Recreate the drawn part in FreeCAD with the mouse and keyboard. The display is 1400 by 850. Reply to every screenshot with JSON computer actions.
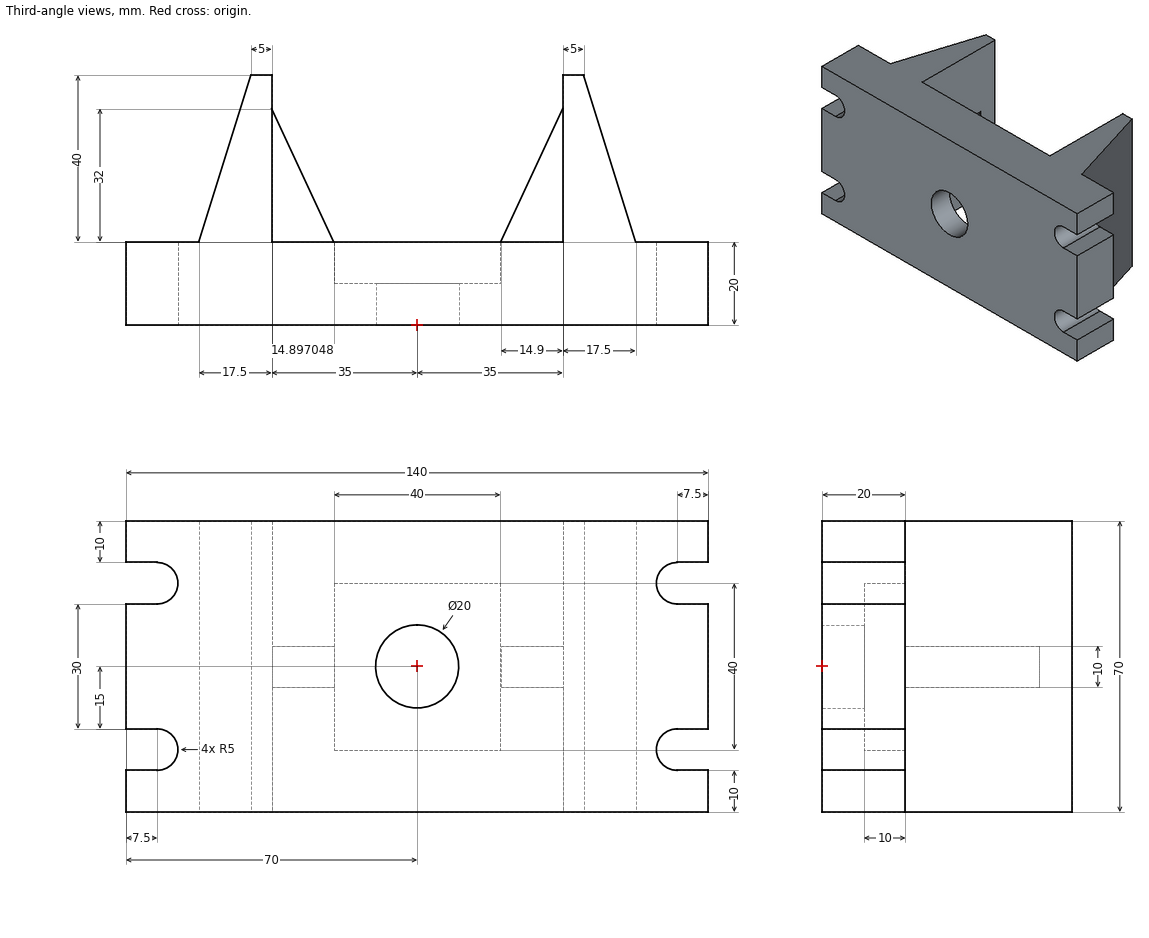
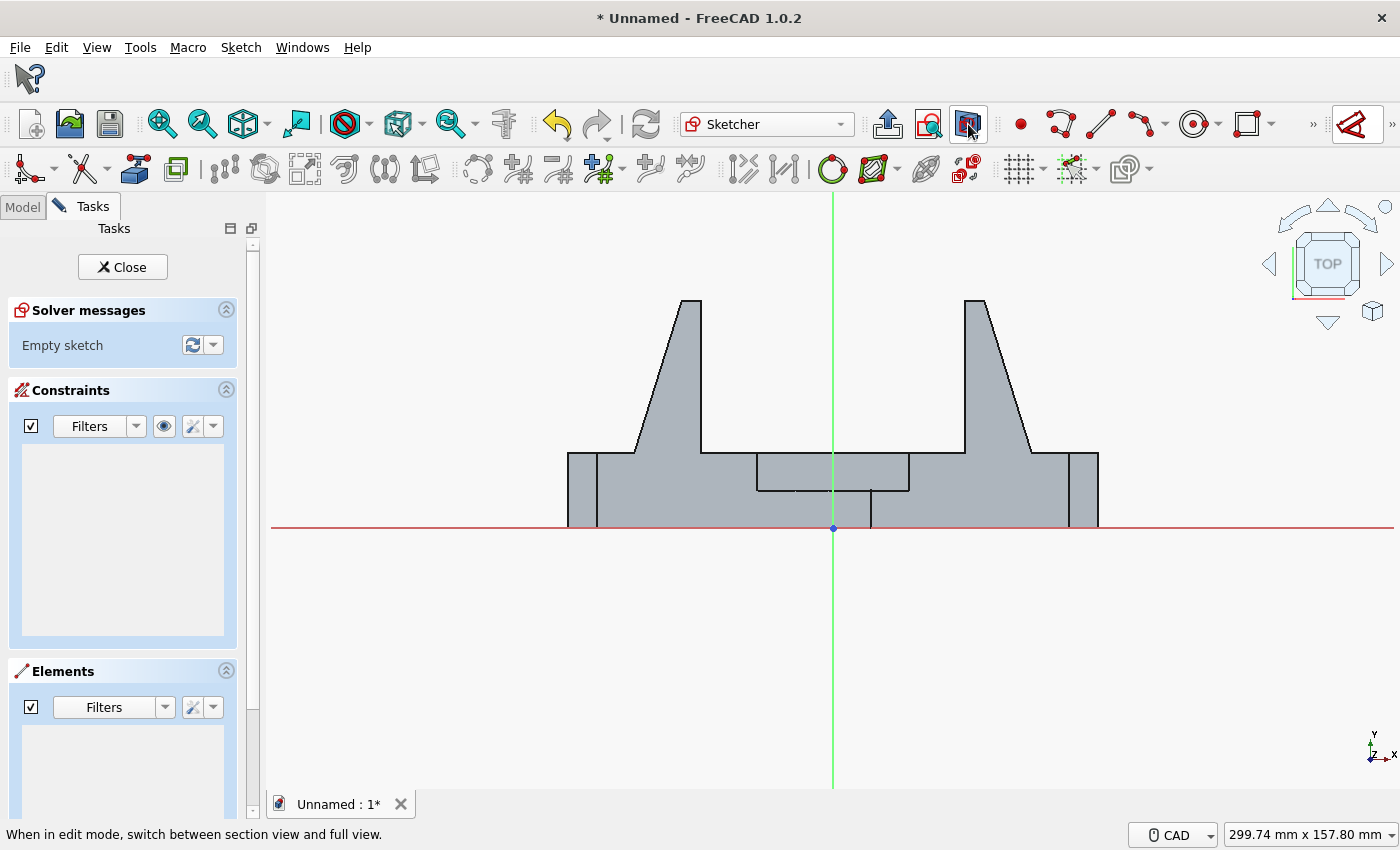
{"action": "scroll", "coordinate": [916, 356], "scroll_direction": "up", "scroll_amount": 3}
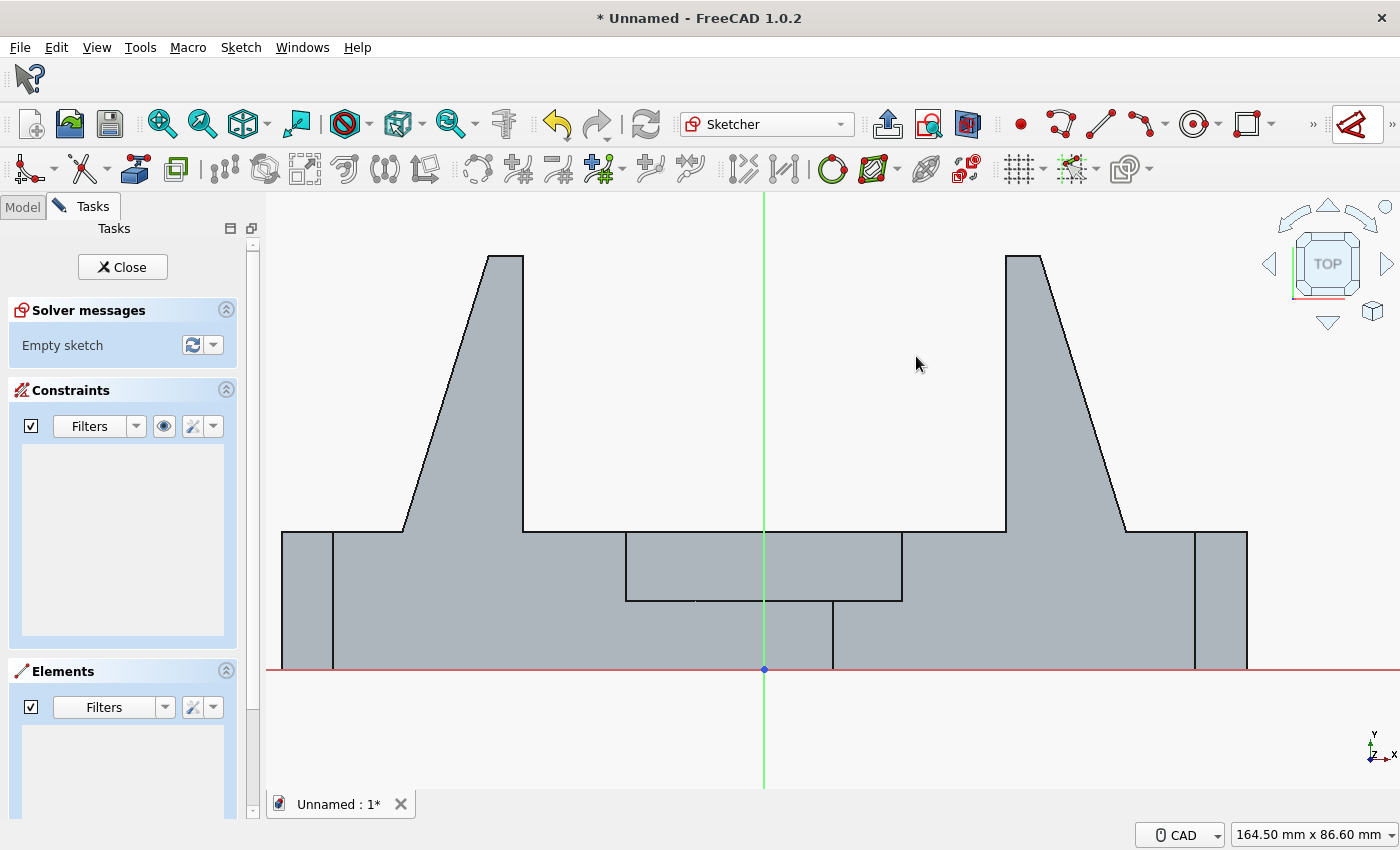
{"action": "left_click", "coordinate": [1062, 124]}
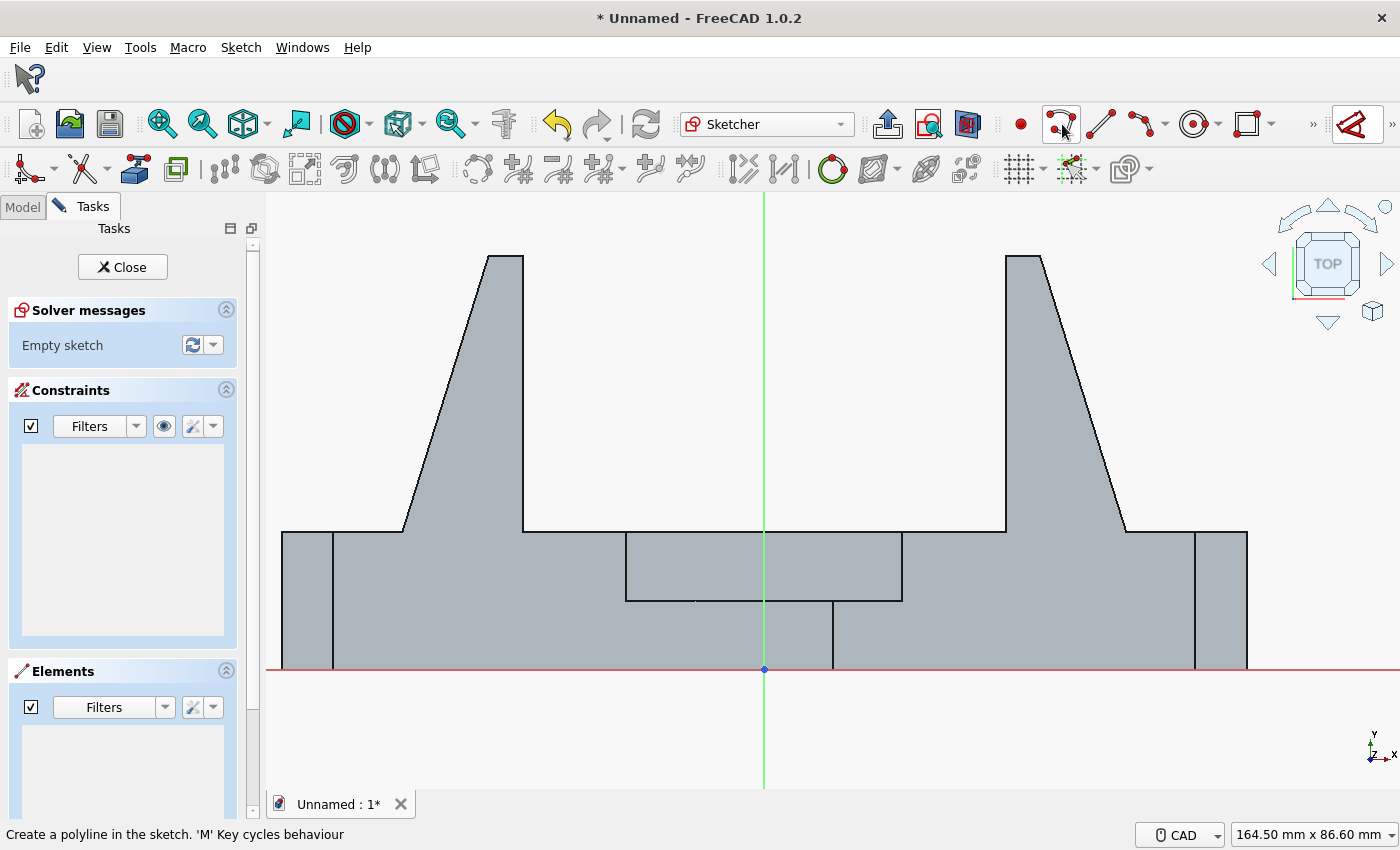
{"action": "left_click", "coordinate": [626, 532]}
{"action": "left_click", "coordinate": [523, 311]}
{"action": "left_click", "coordinate": [523, 532]}
{"action": "left_click", "coordinate": [626, 533]}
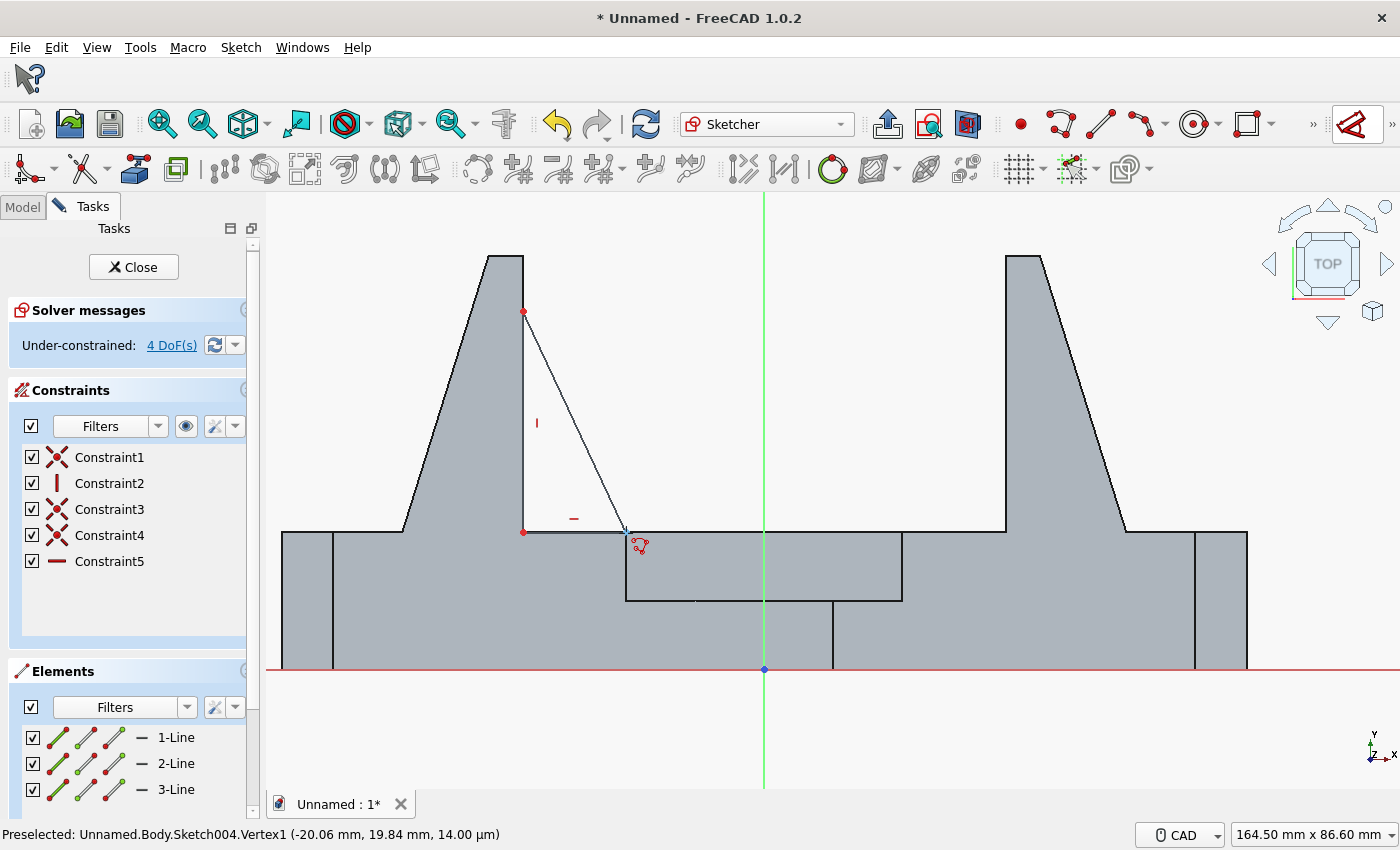
{"action": "left_click", "coordinate": [903, 532]}
{"action": "left_click", "coordinate": [1006, 532]}
{"action": "left_click", "coordinate": [1006, 311]}
{"action": "left_click", "coordinate": [903, 533]}
{"action": "key", "text": "Escape"}
{"action": "key", "text": "Escape"}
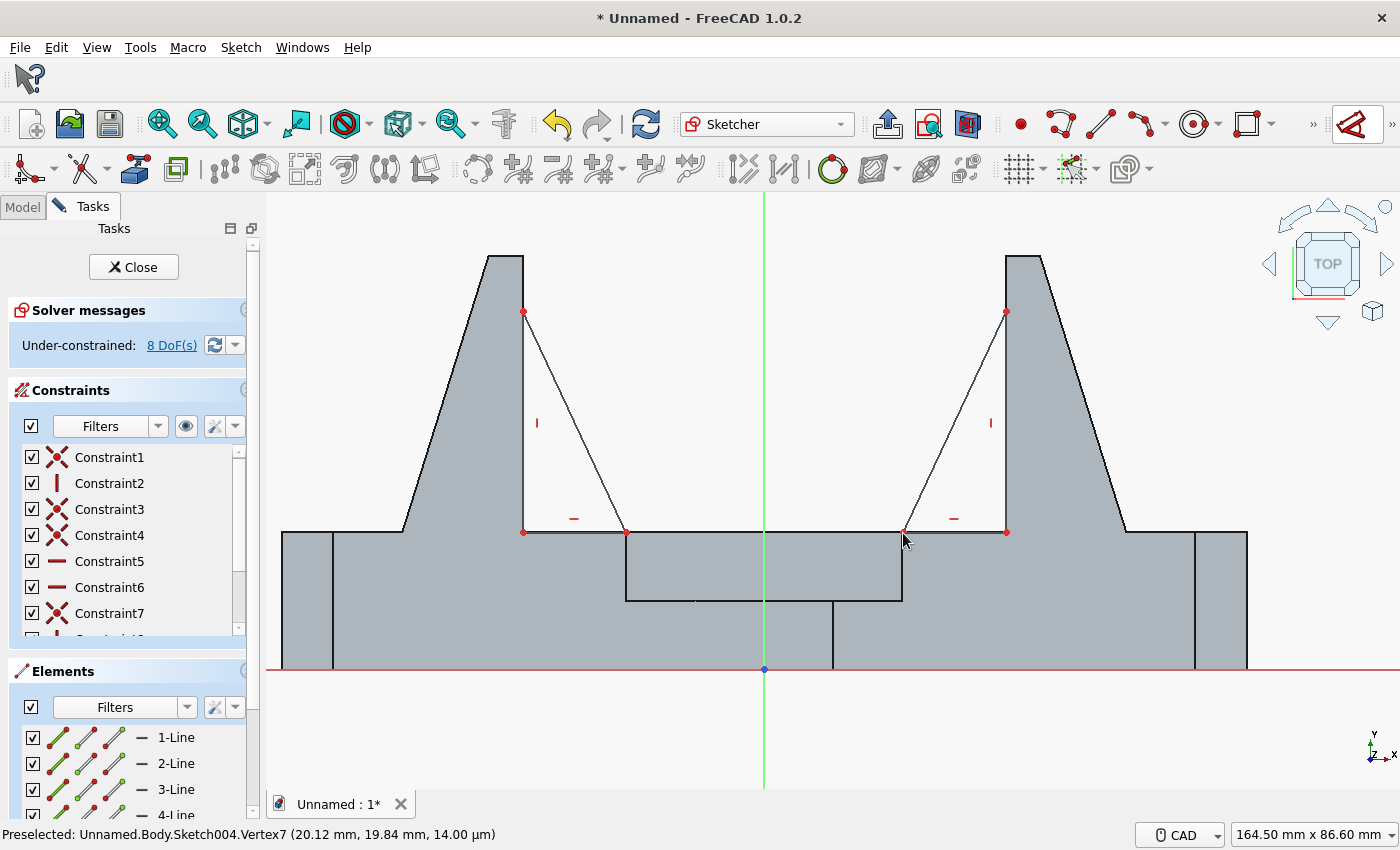
{"action": "left_click", "coordinate": [523, 378]}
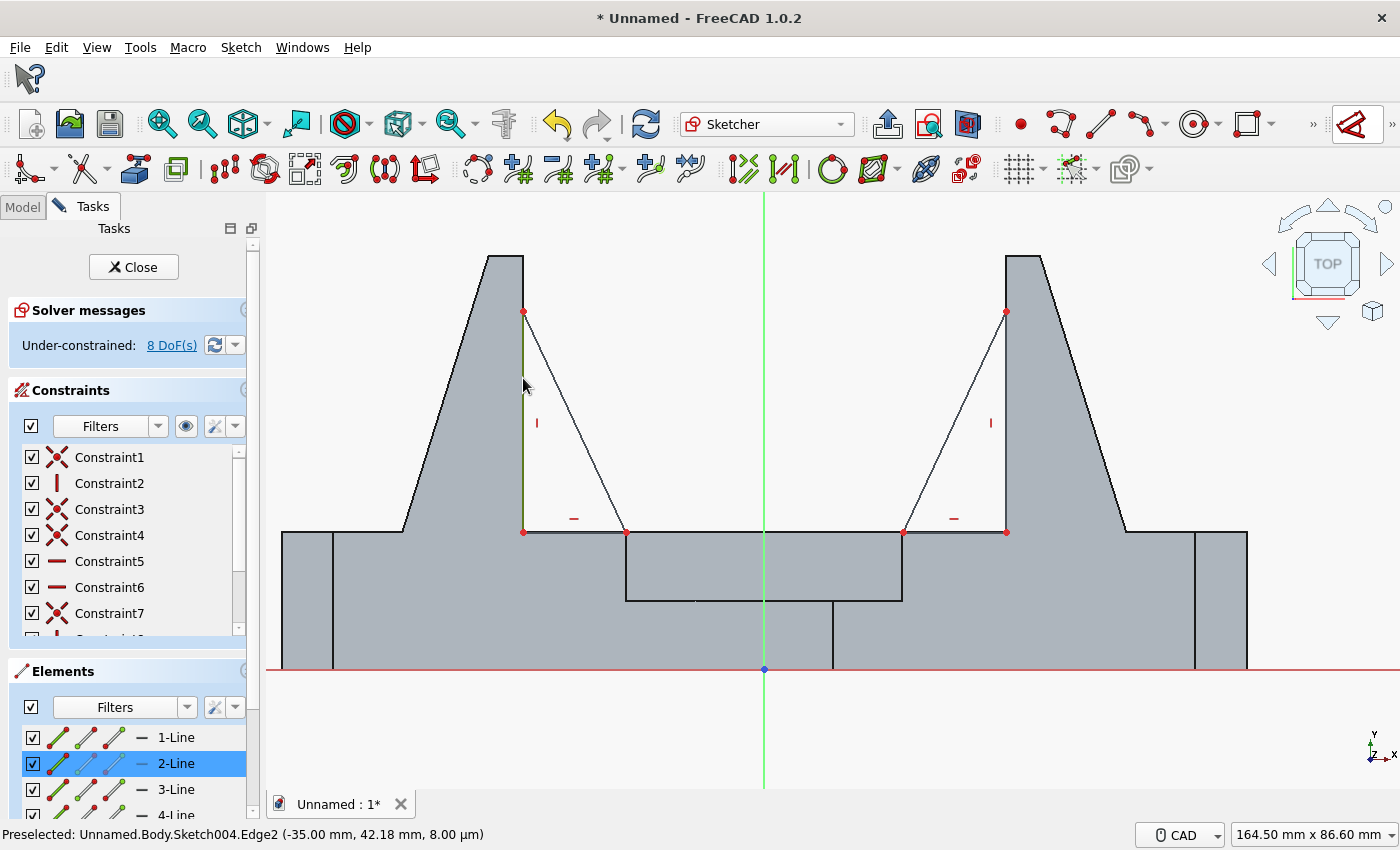
{"action": "key", "text": "i"}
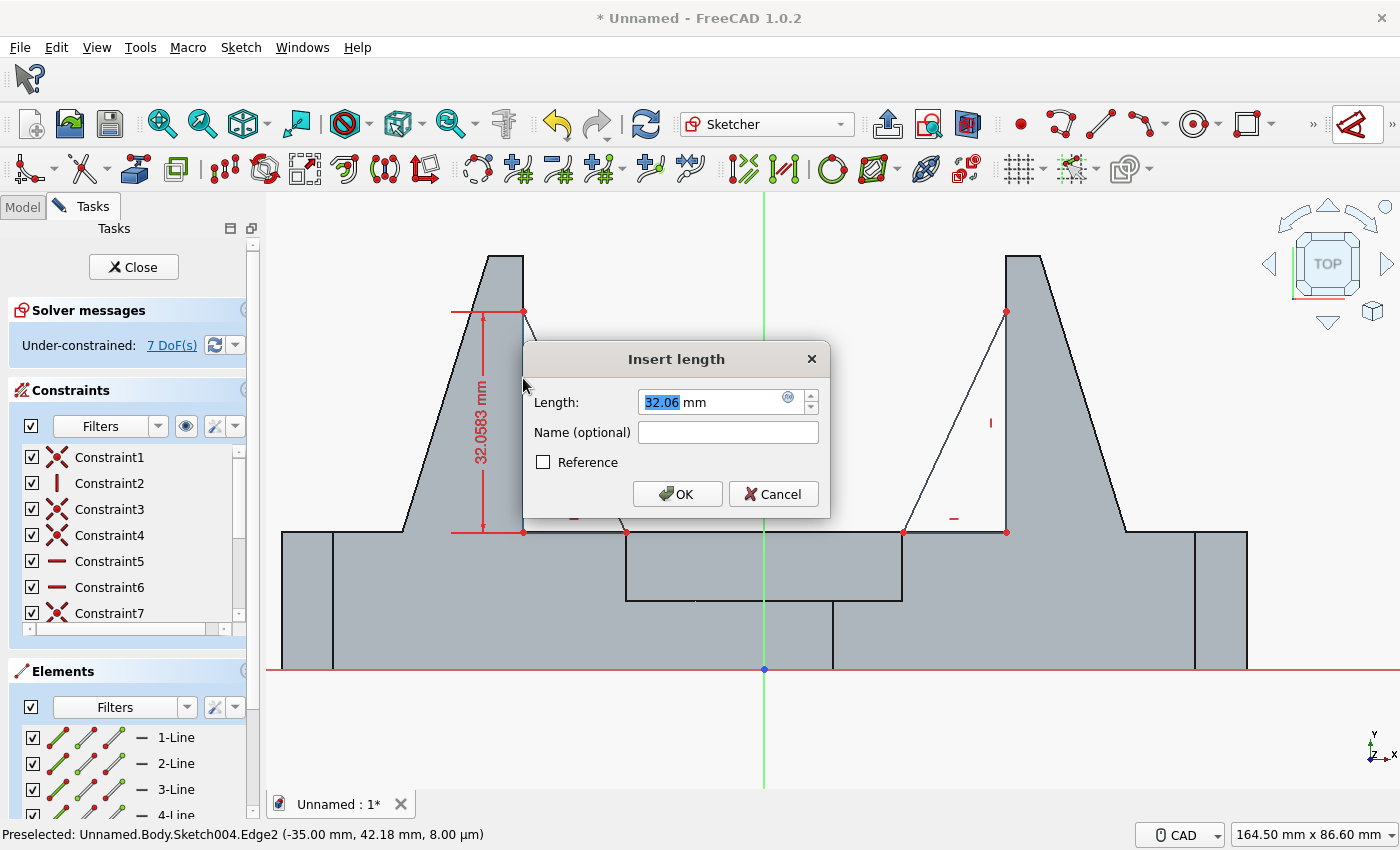
{"action": "type", "text": "32"}
{"action": "key", "text": "Return"}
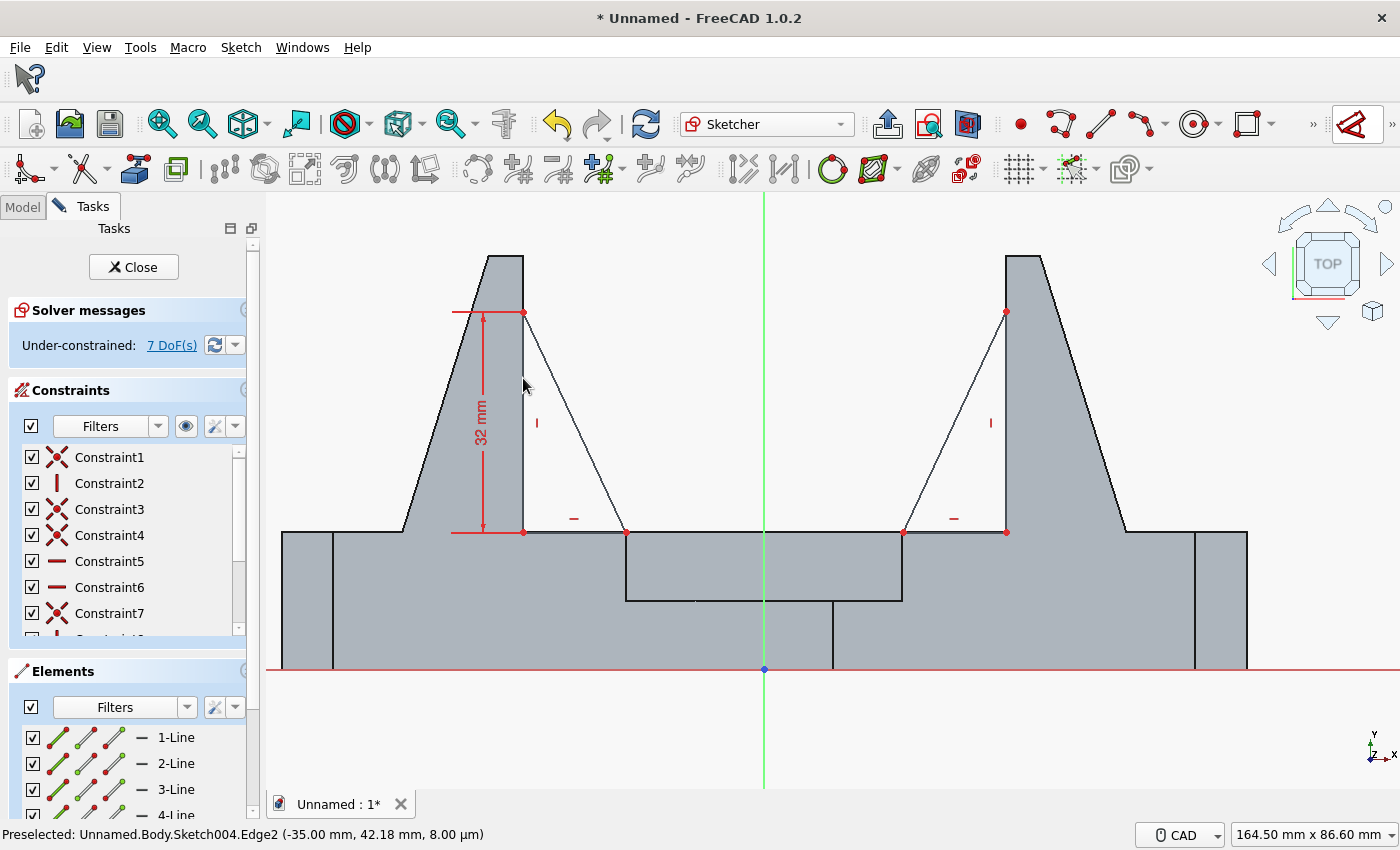
{"action": "left_click", "coordinate": [1006, 467]}